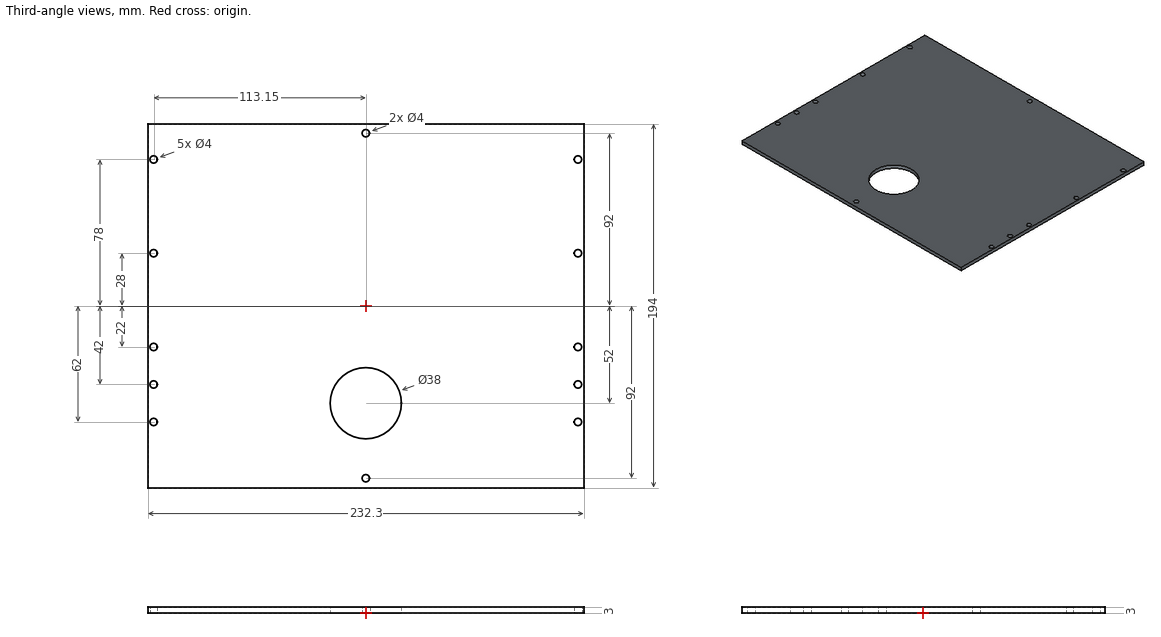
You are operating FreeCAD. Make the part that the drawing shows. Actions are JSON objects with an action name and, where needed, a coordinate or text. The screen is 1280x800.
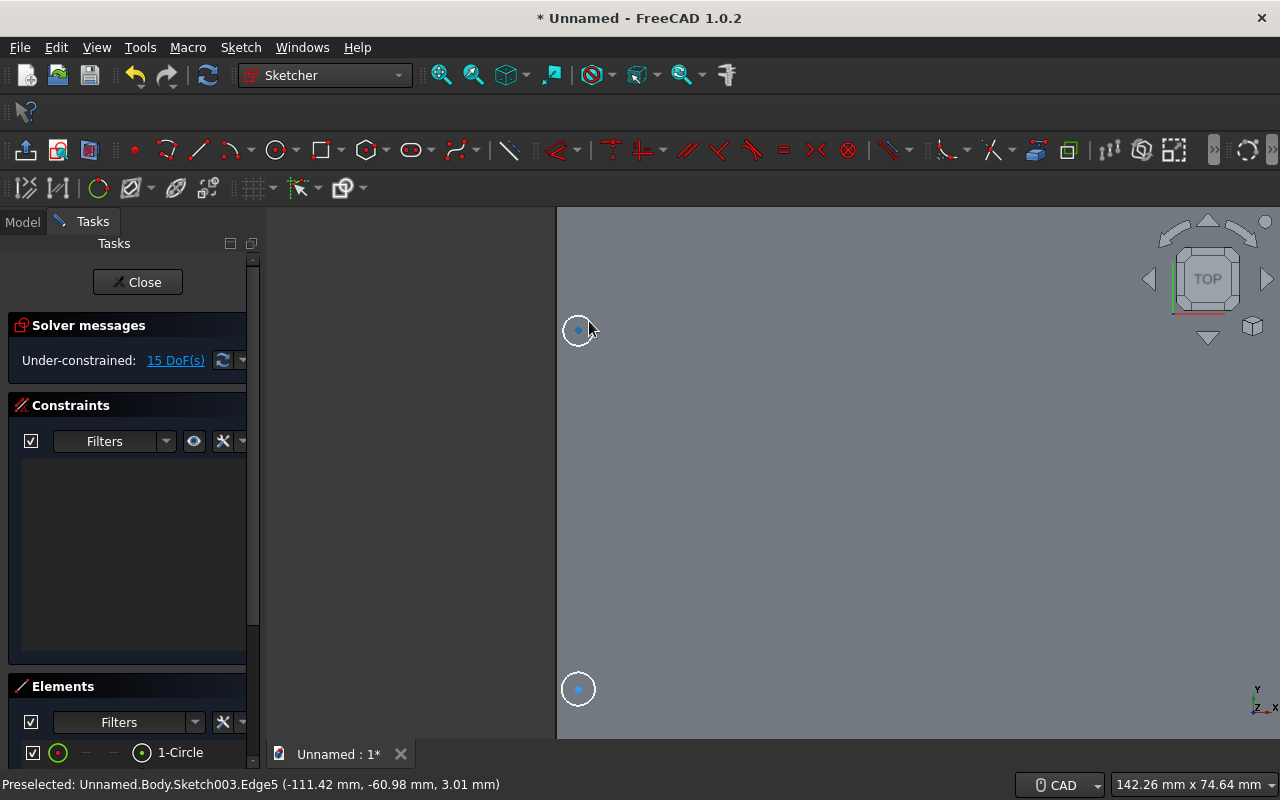
{"action": "left_click", "coordinate": [589, 320]}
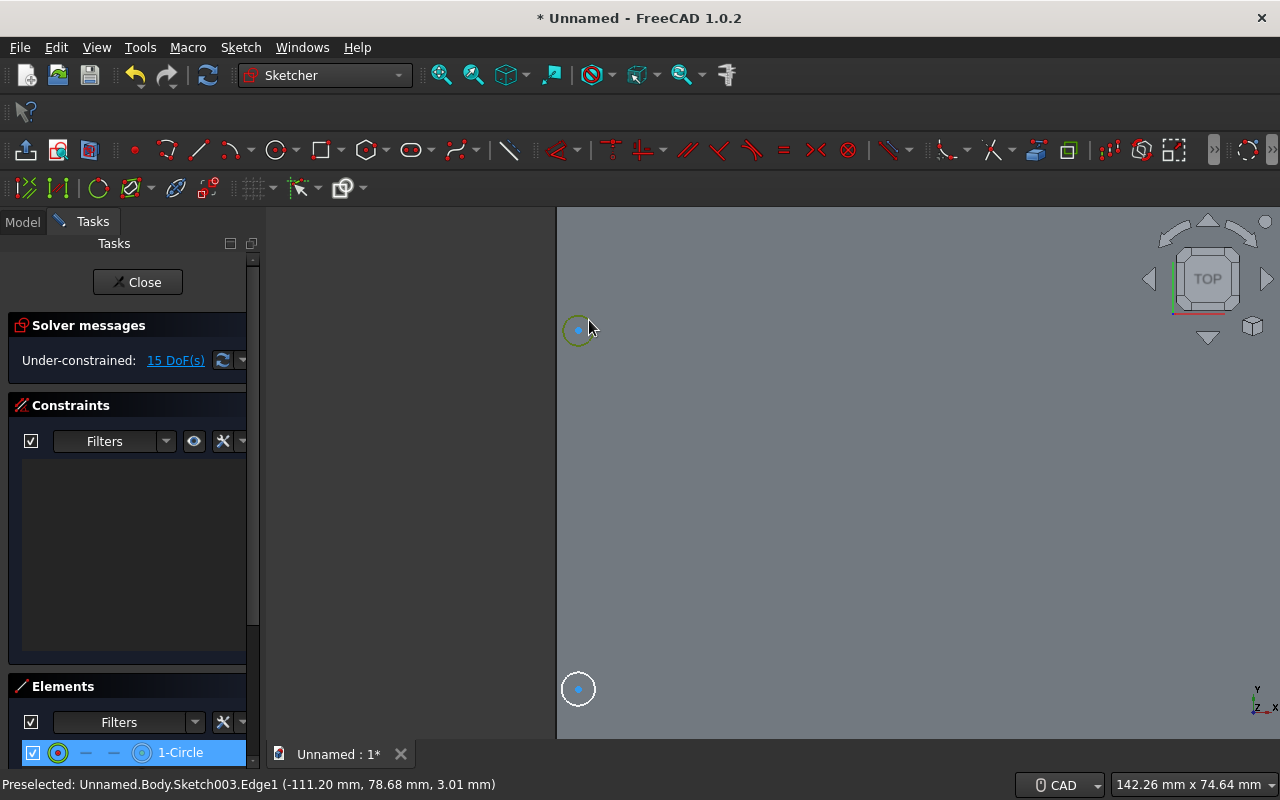
{"action": "left_click", "coordinate": [590, 677]}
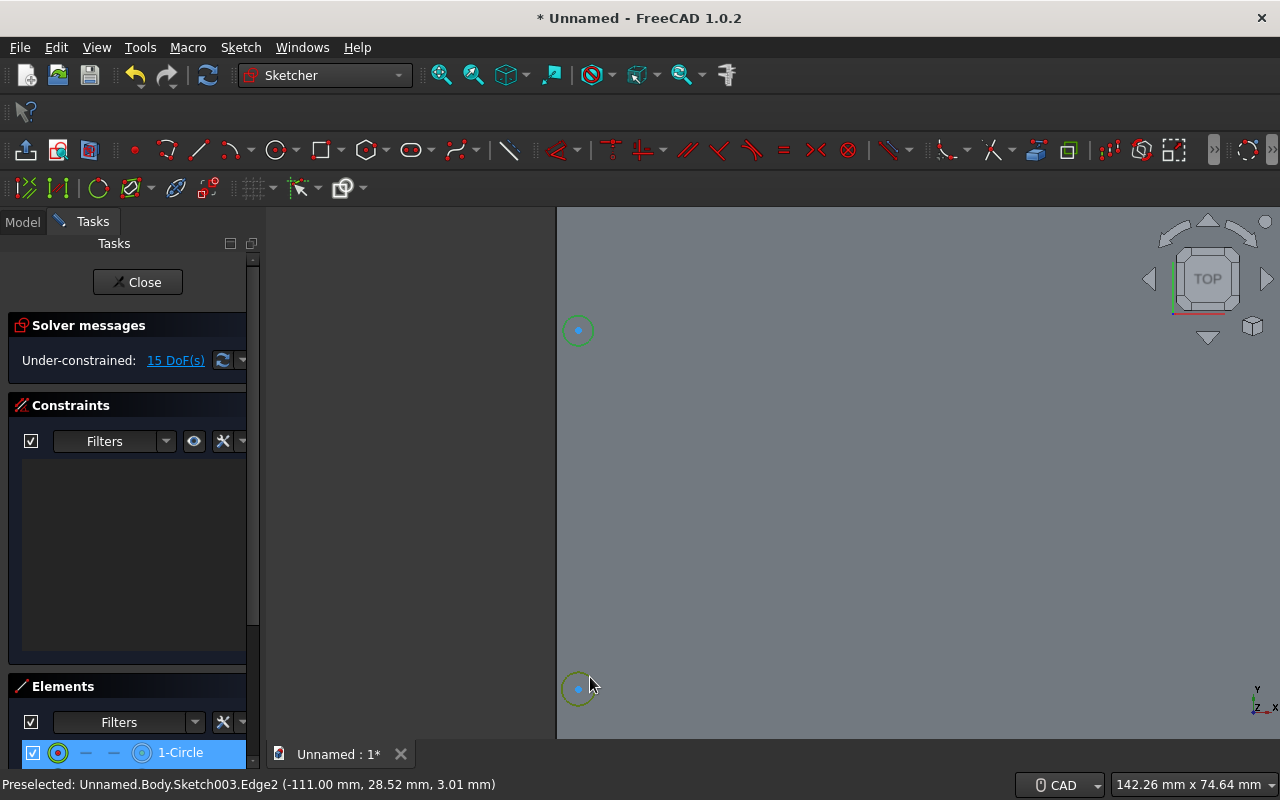
{"action": "scroll", "coordinate": [588, 320], "scroll_direction": "down", "scroll_amount": 6}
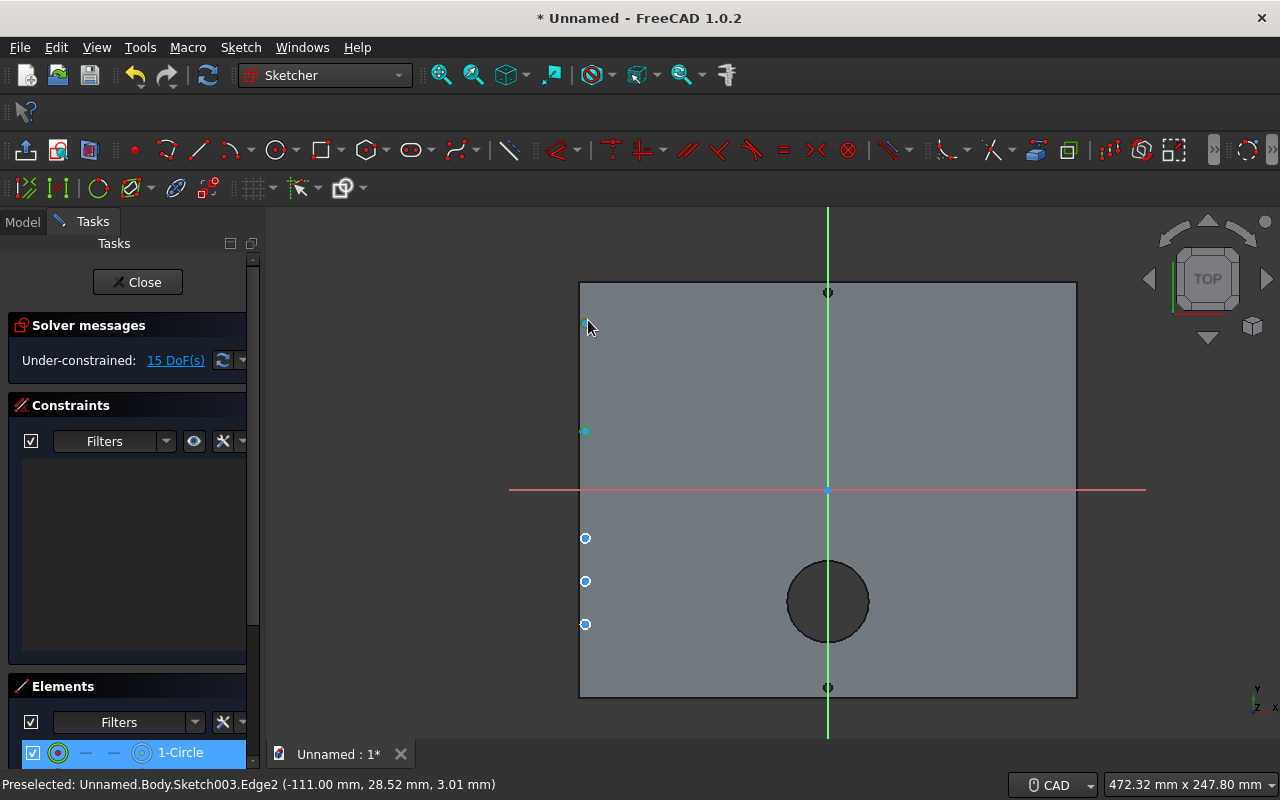
{"action": "scroll", "coordinate": [589, 535], "scroll_direction": "up", "scroll_amount": 6}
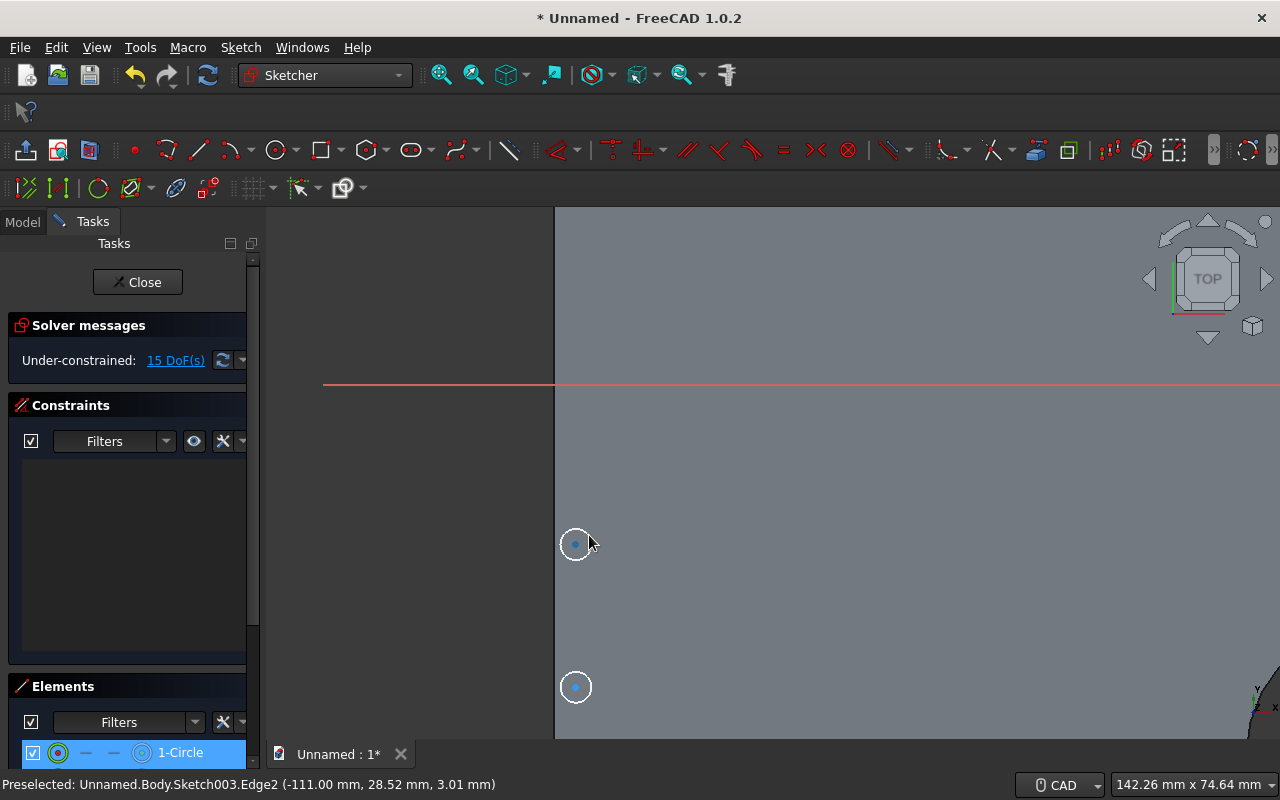
{"action": "left_click", "coordinate": [587, 534]}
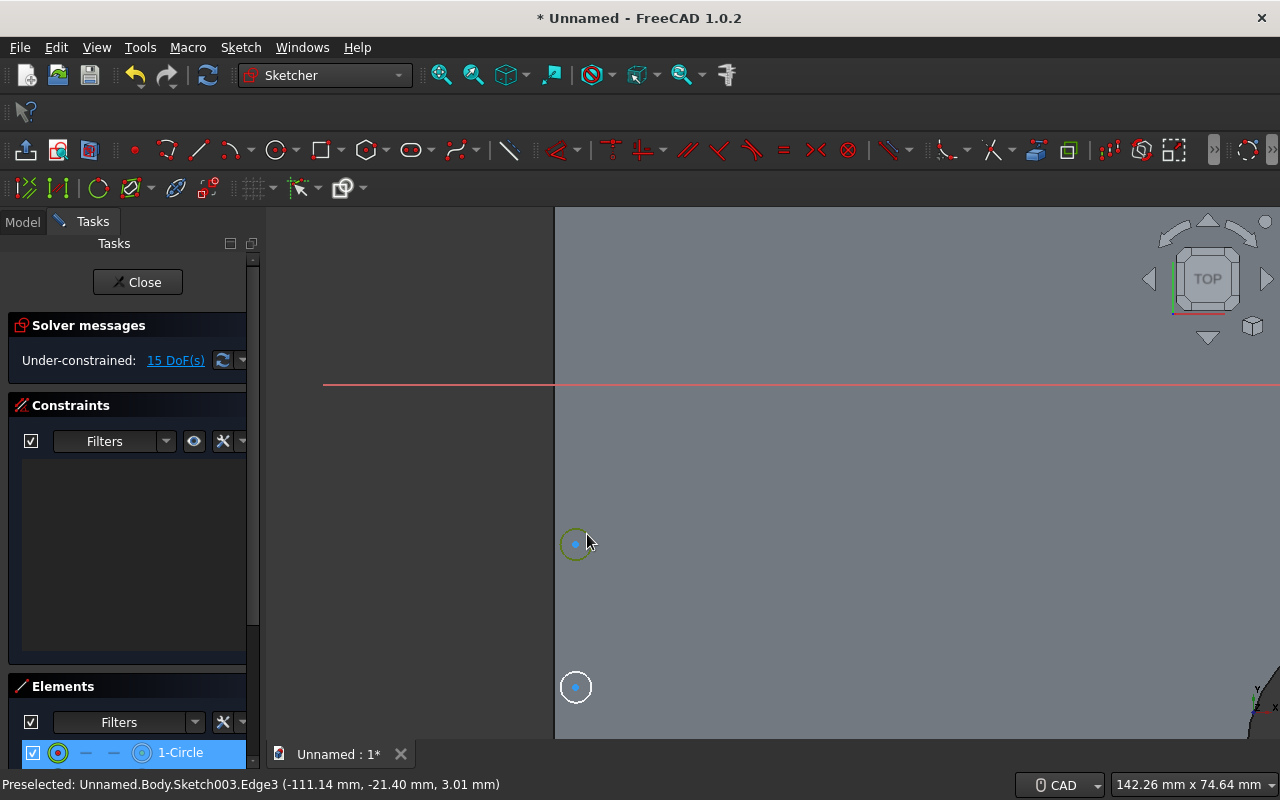
{"action": "left_click", "coordinate": [587, 676]}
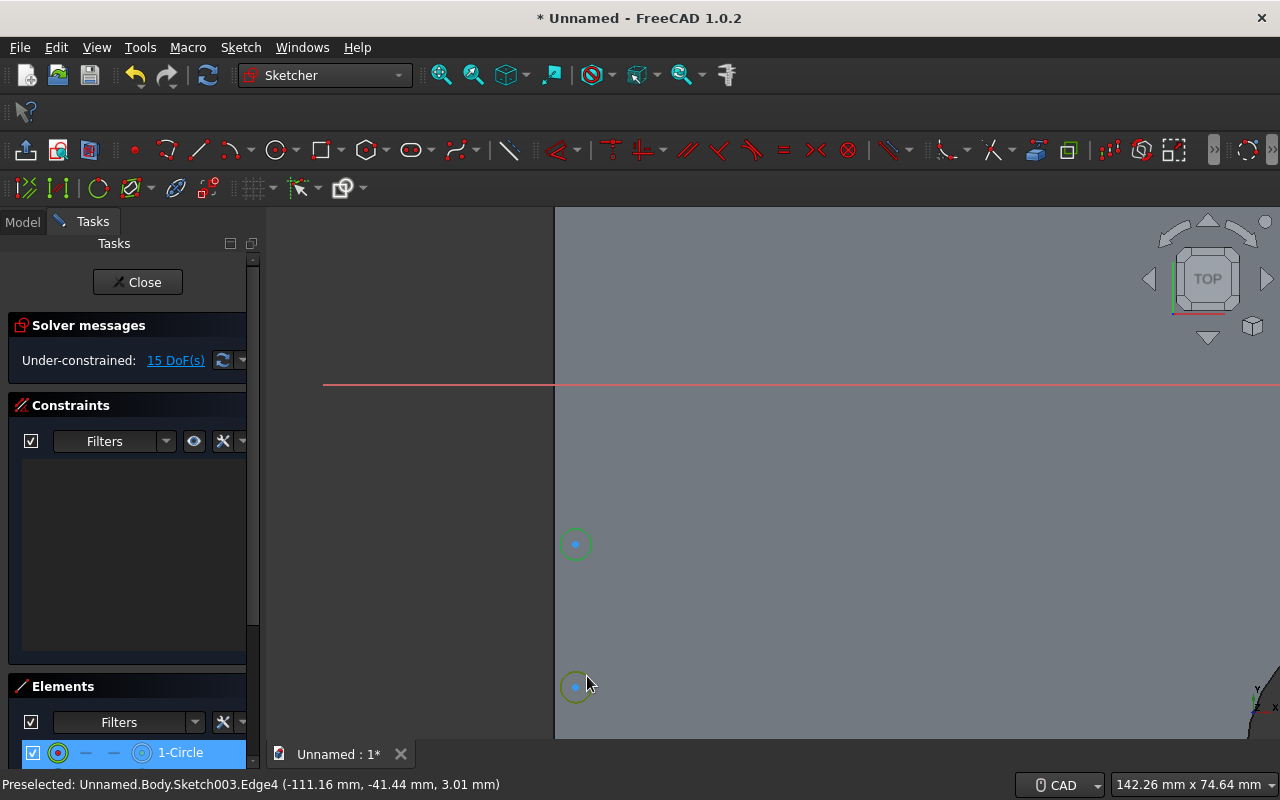
{"action": "scroll", "coordinate": [589, 536], "scroll_direction": "down", "scroll_amount": 6}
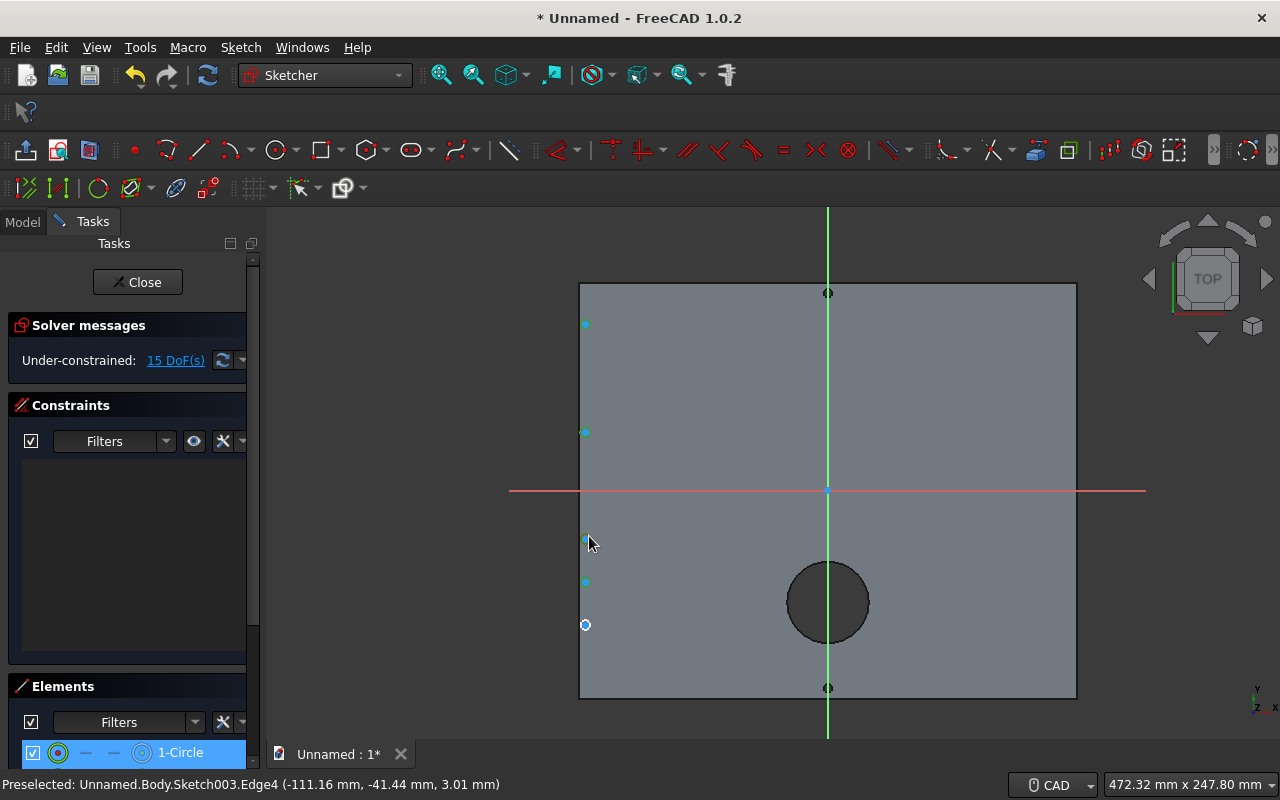
{"action": "scroll", "coordinate": [589, 622], "scroll_direction": "up", "scroll_amount": 6}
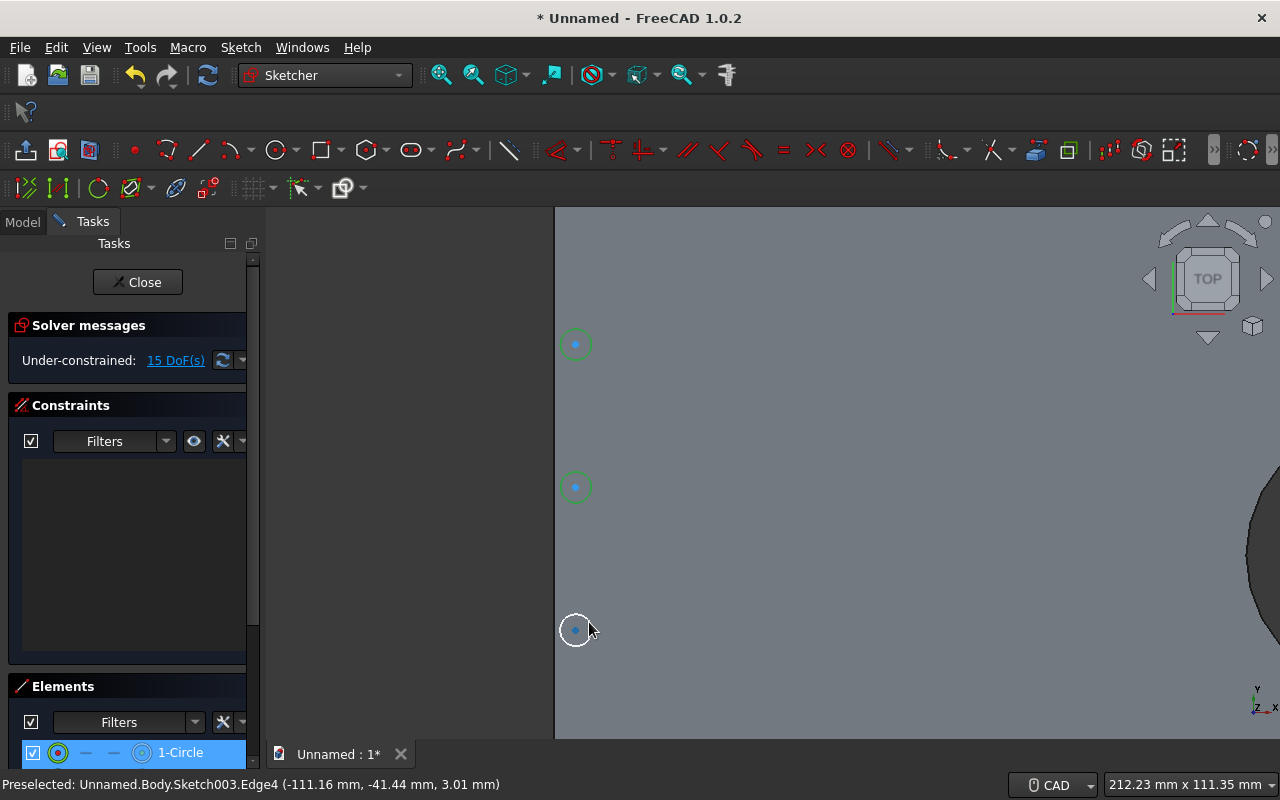
{"action": "left_click", "coordinate": [587, 619]}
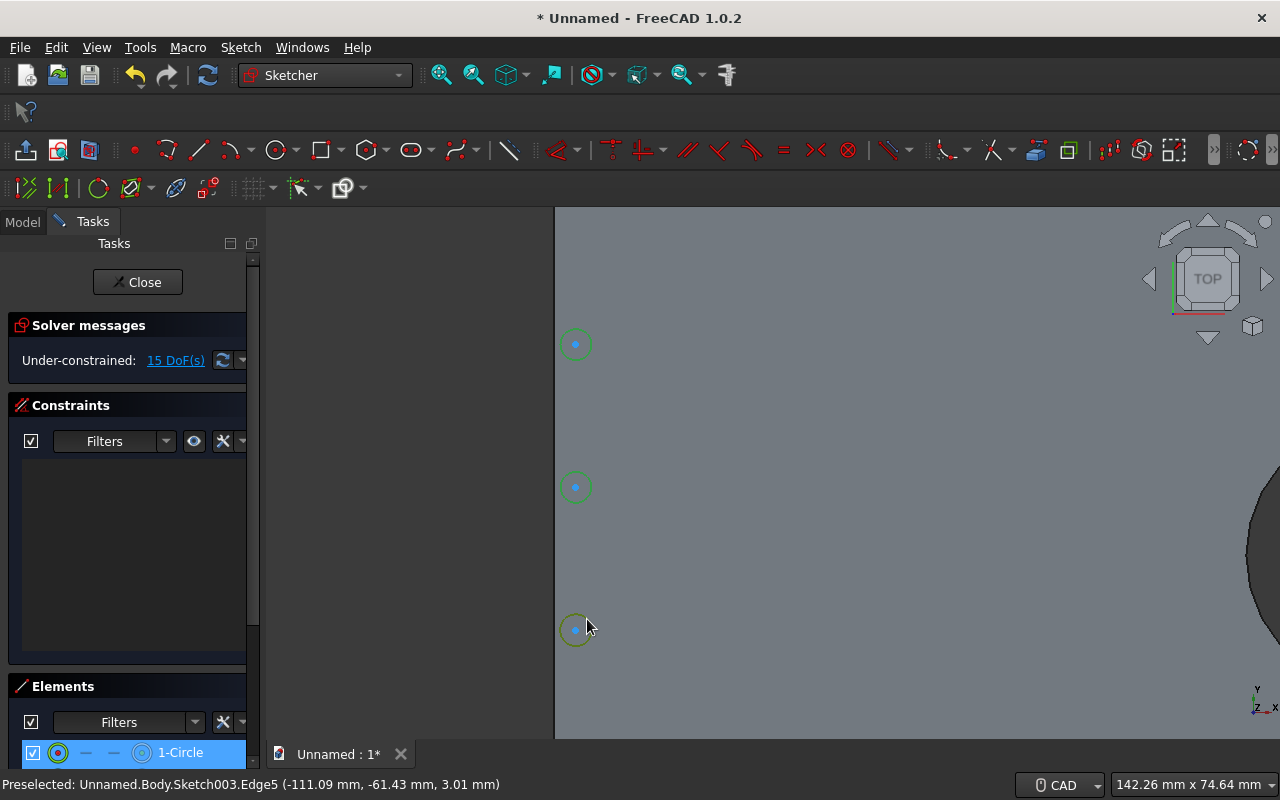
{"action": "key", "text": "e"}